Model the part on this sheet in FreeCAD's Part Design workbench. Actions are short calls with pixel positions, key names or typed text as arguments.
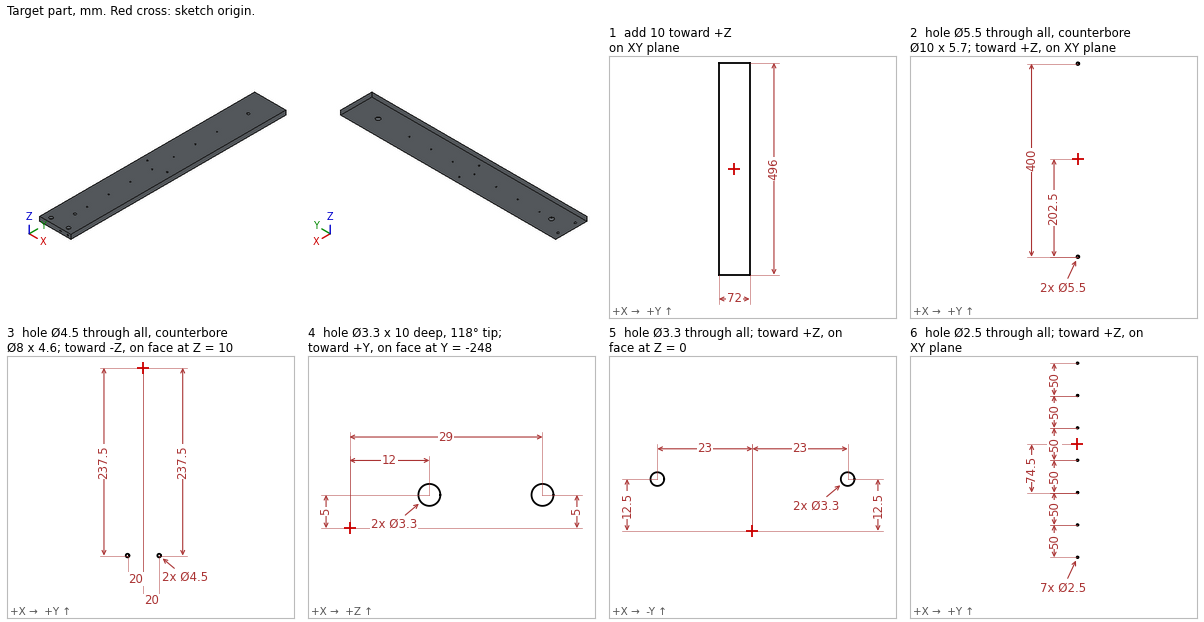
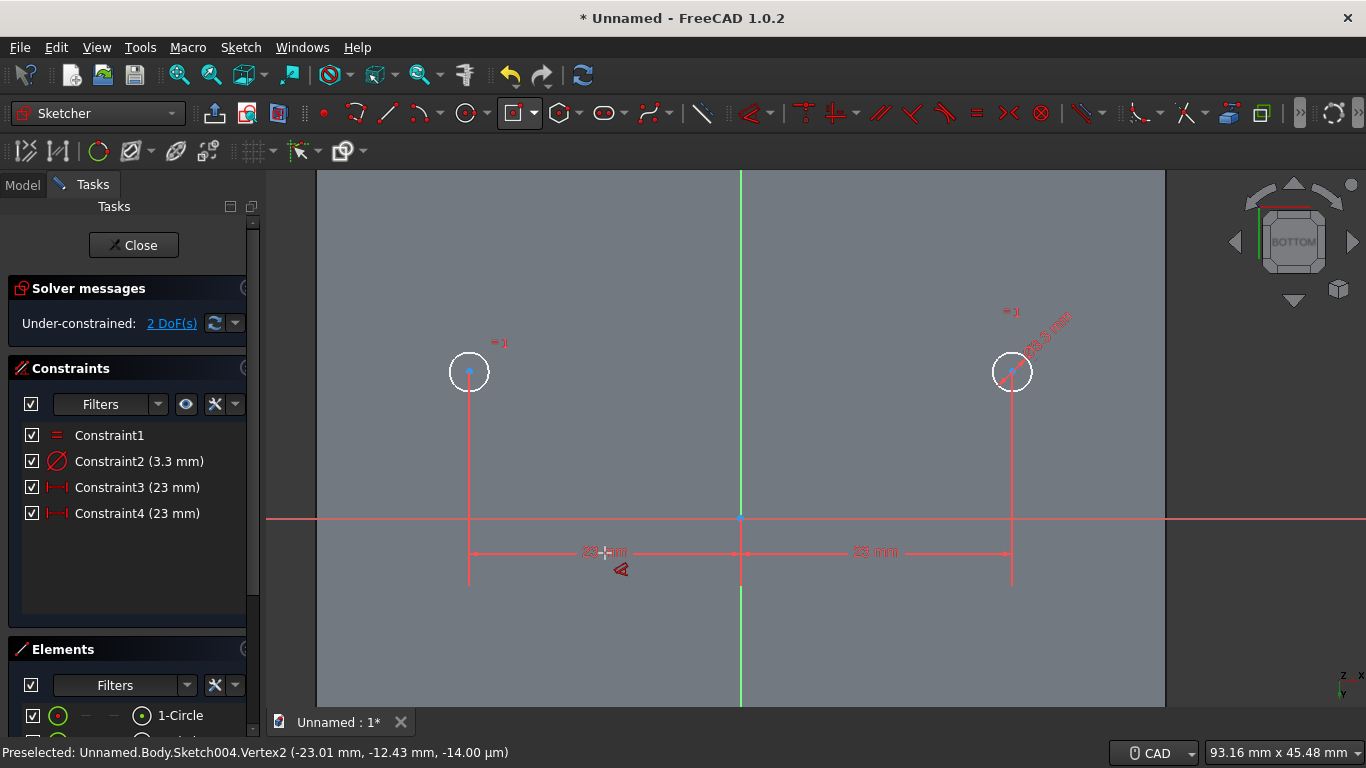
click(1012, 372)
click(1046, 445)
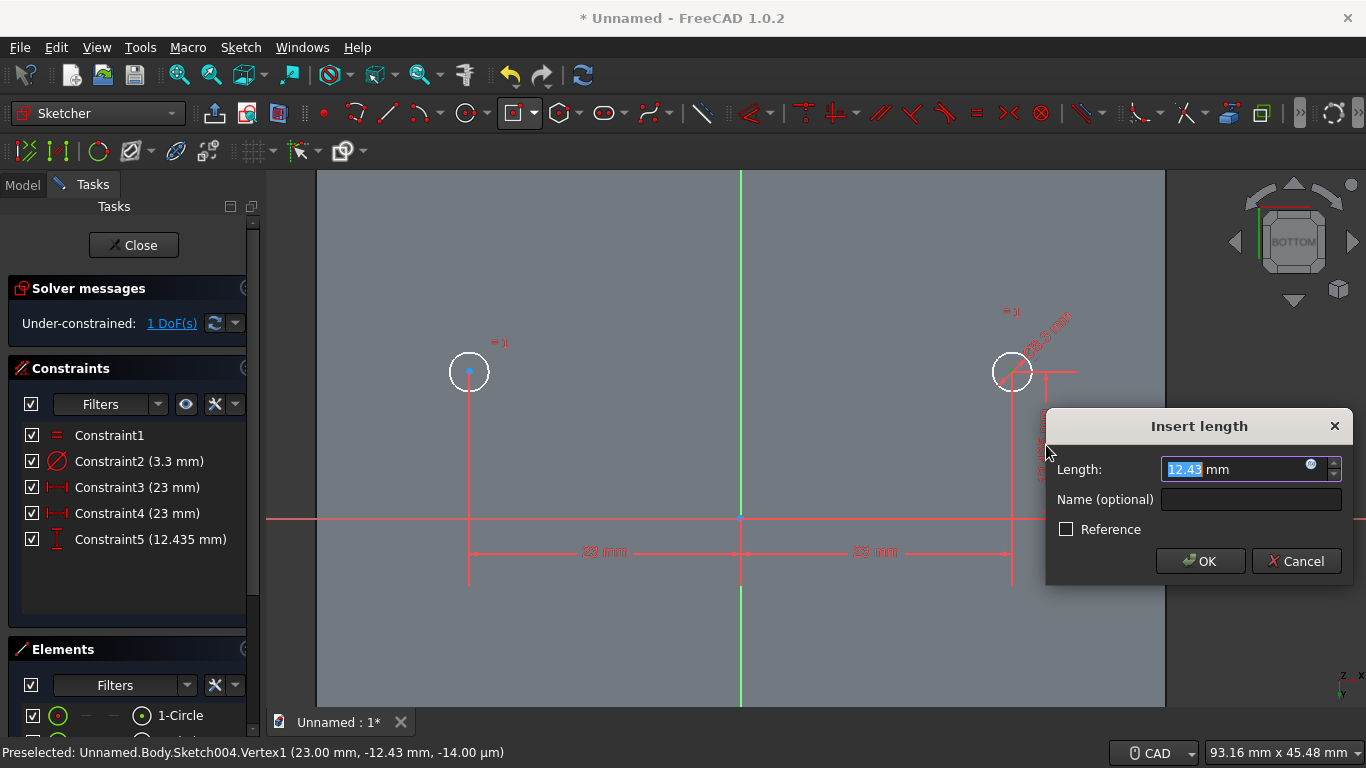
text(12.5)
key(Return)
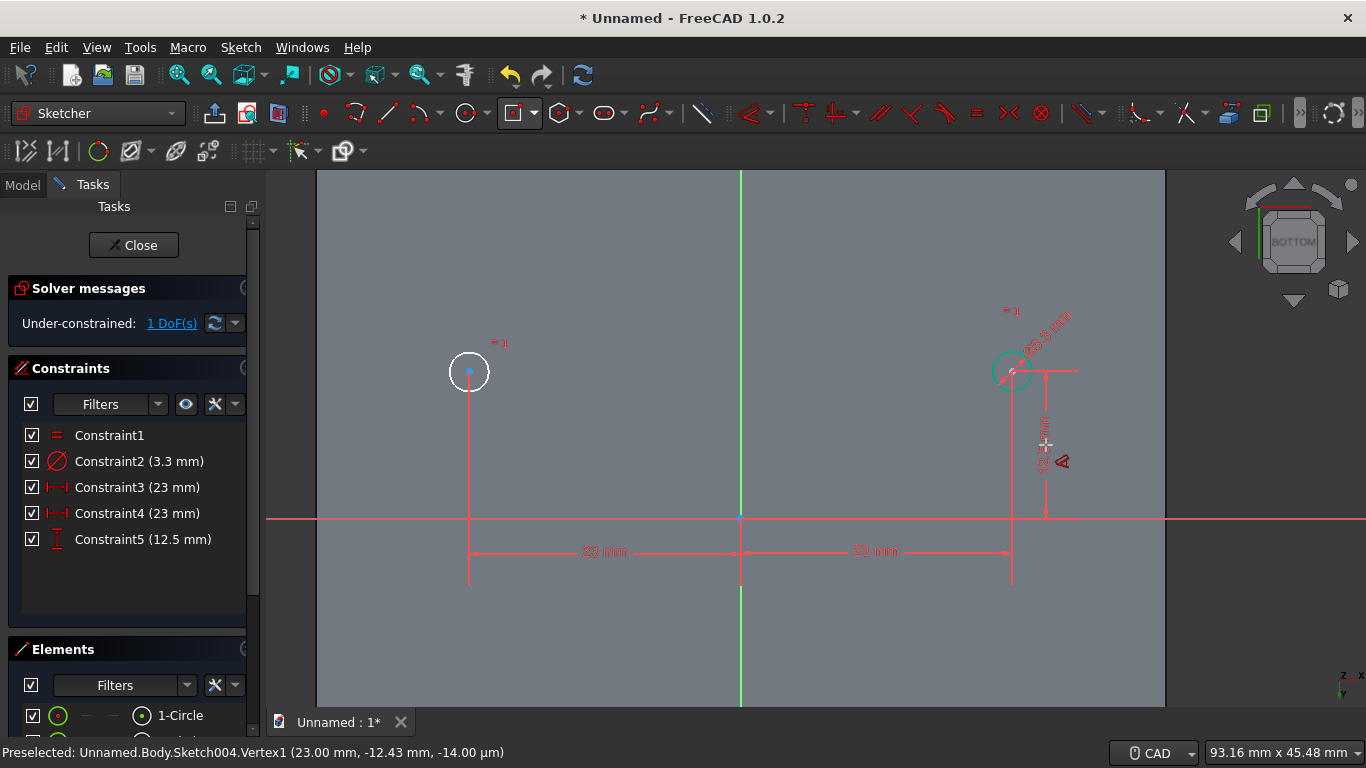
click(469, 372)
click(435, 445)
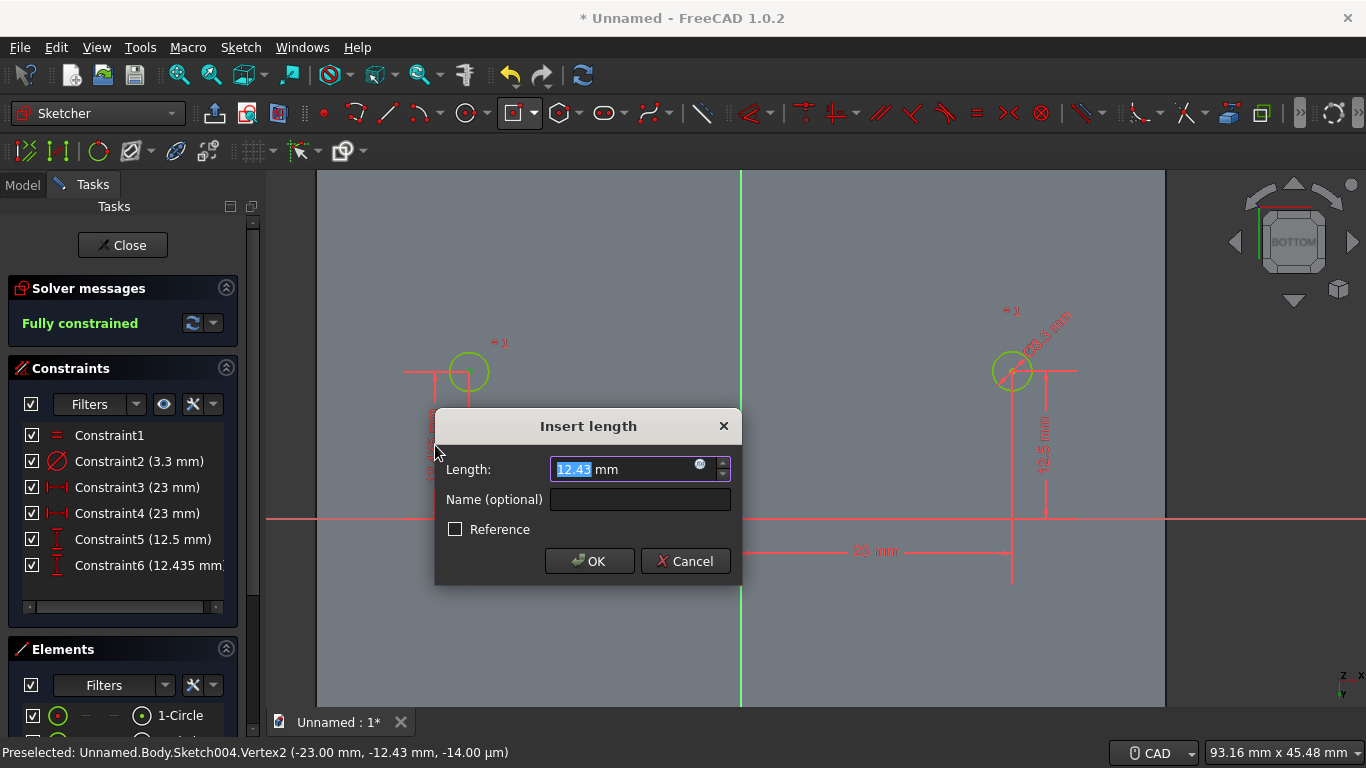
text(12.5)
key(Return)
key(Escape)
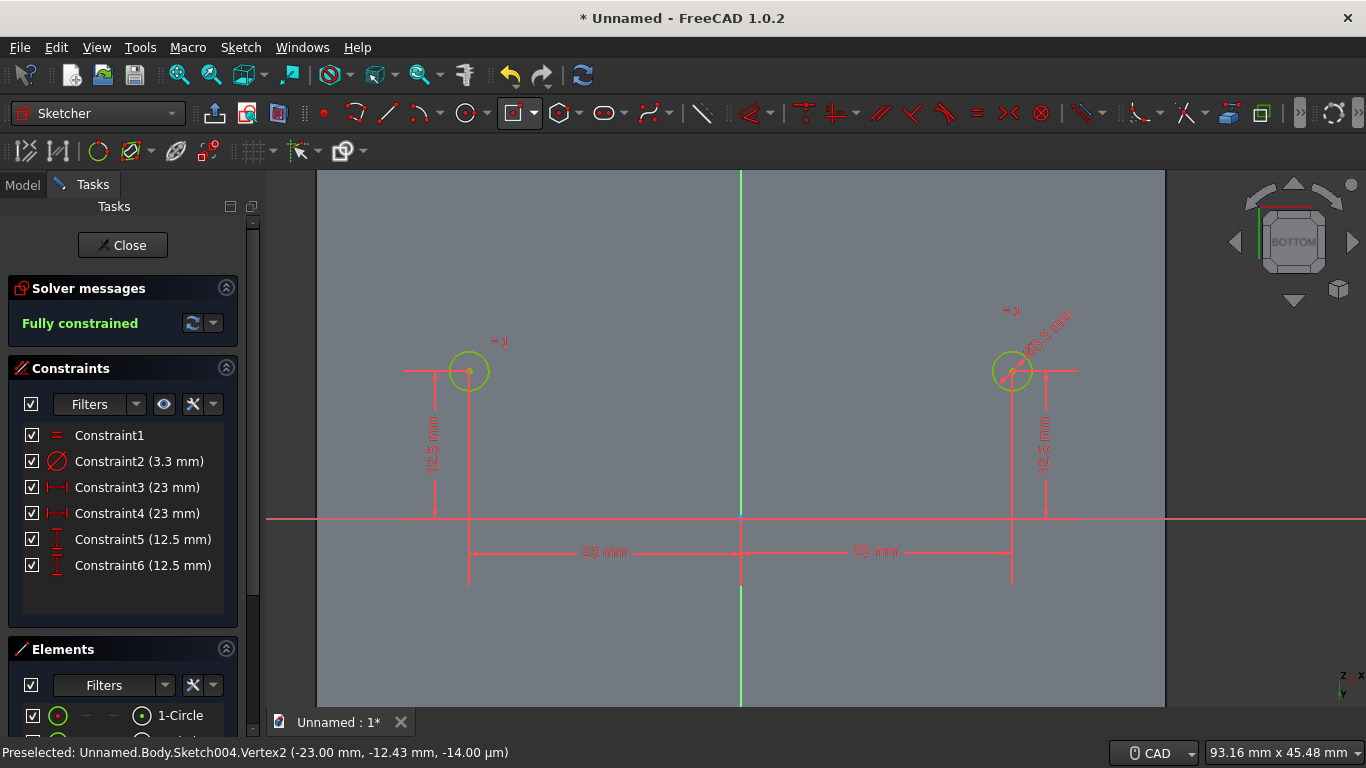
click(123, 245)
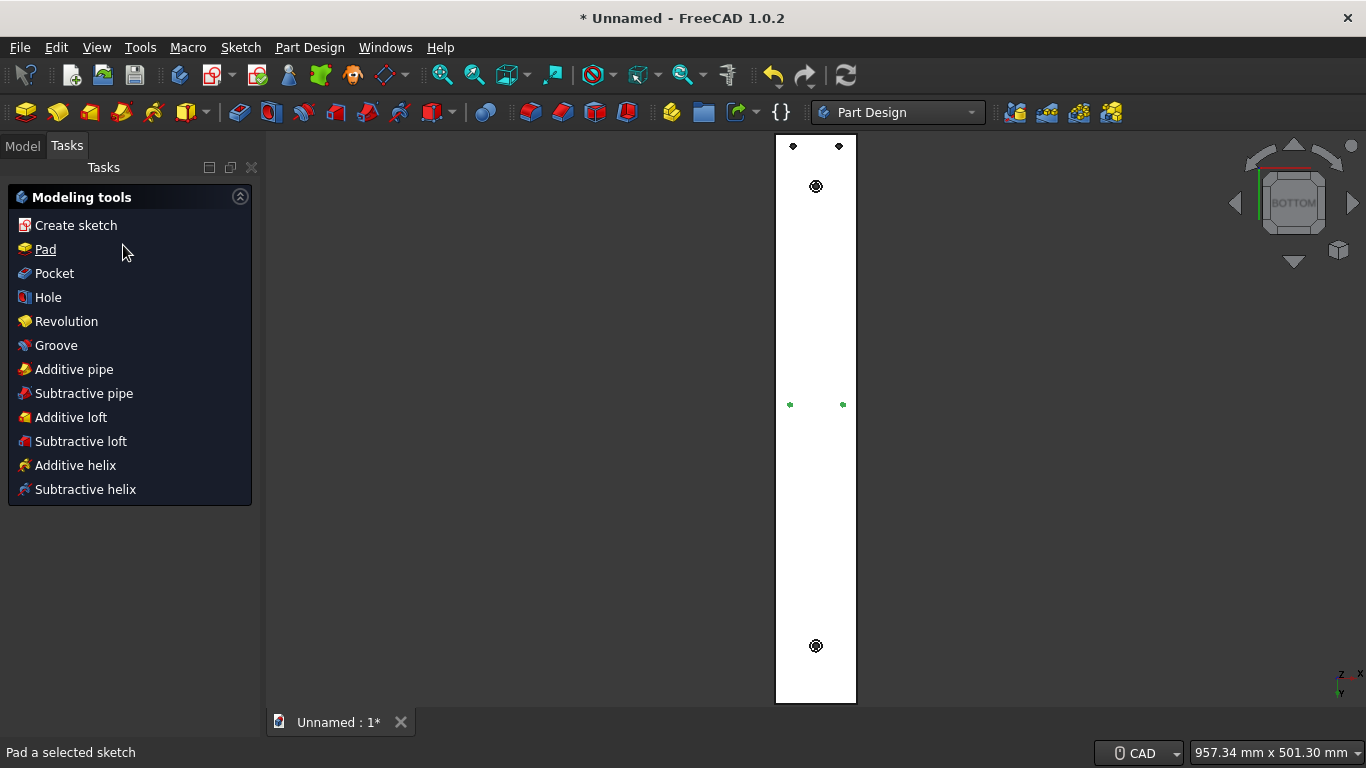
click(272, 112)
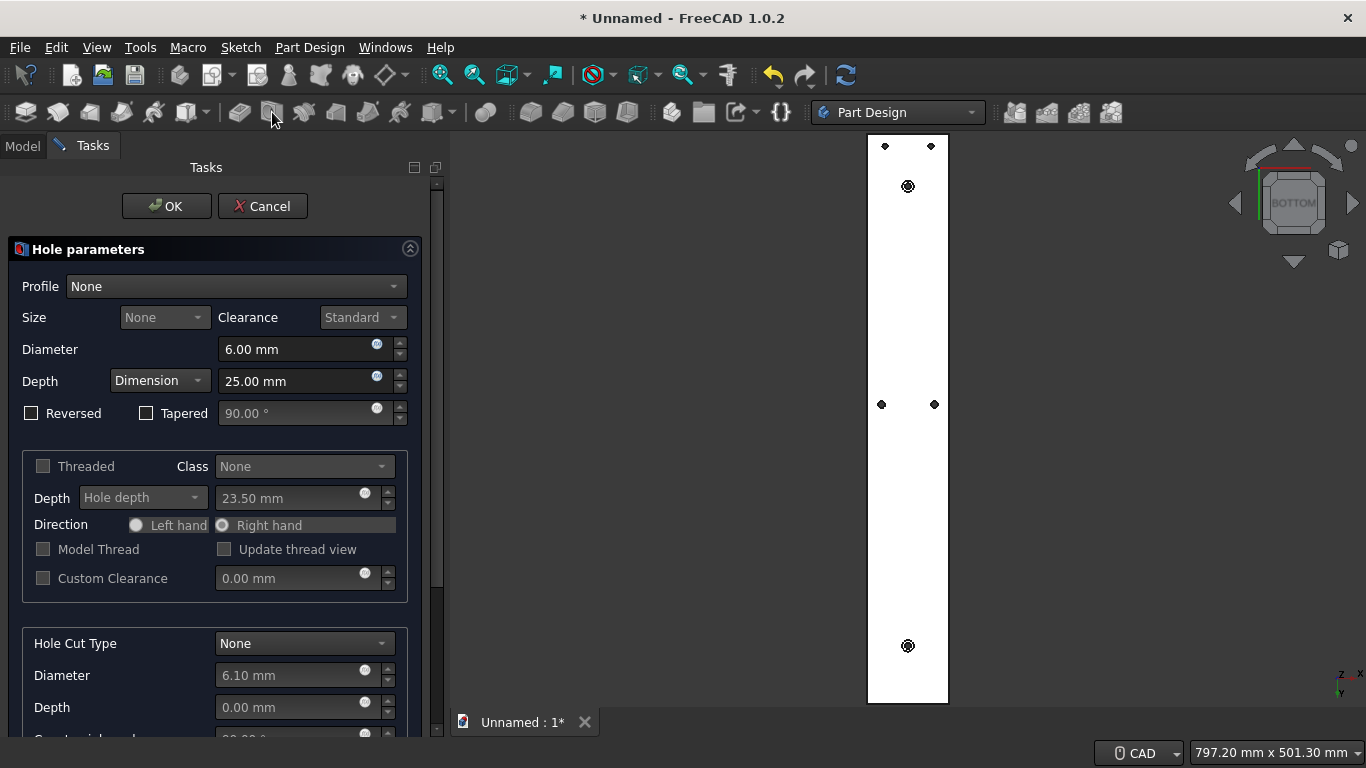
triple_click(305, 349)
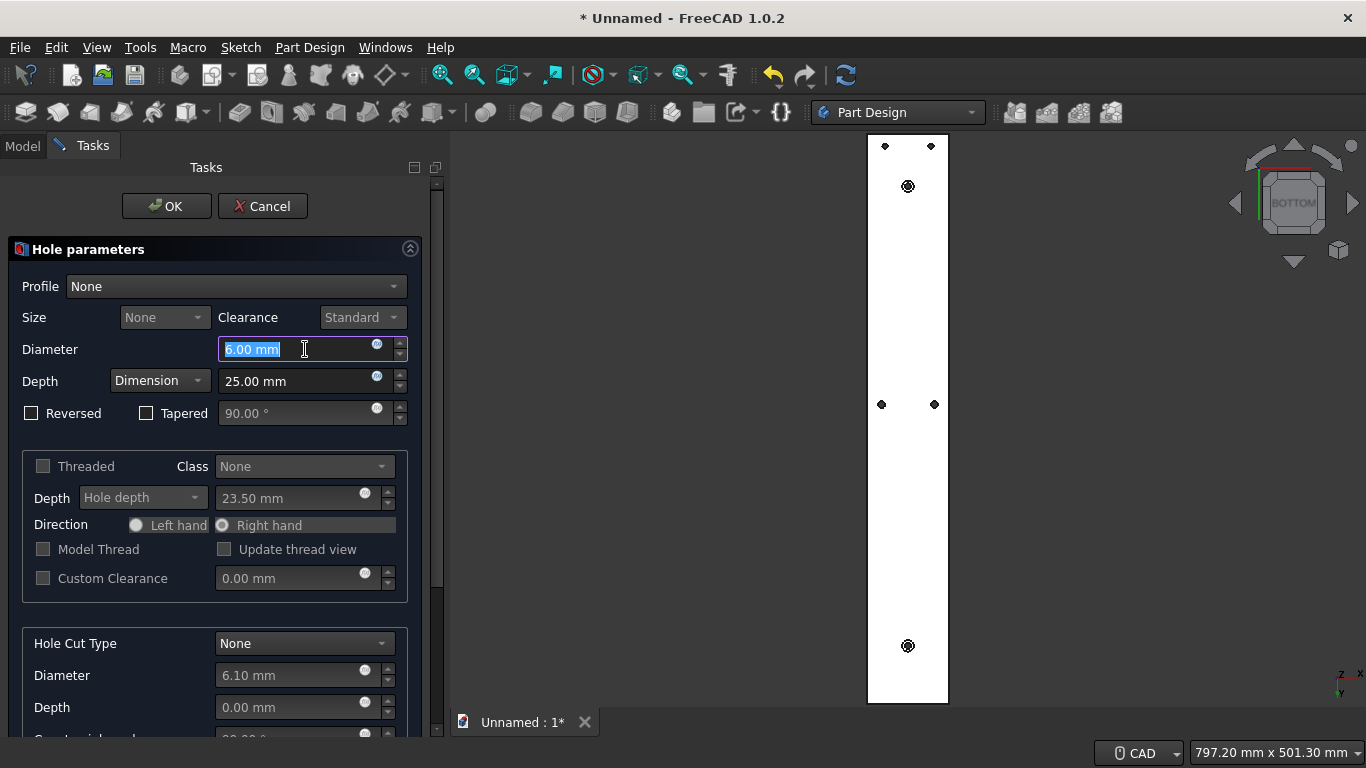
text(3.3)
key(Tab)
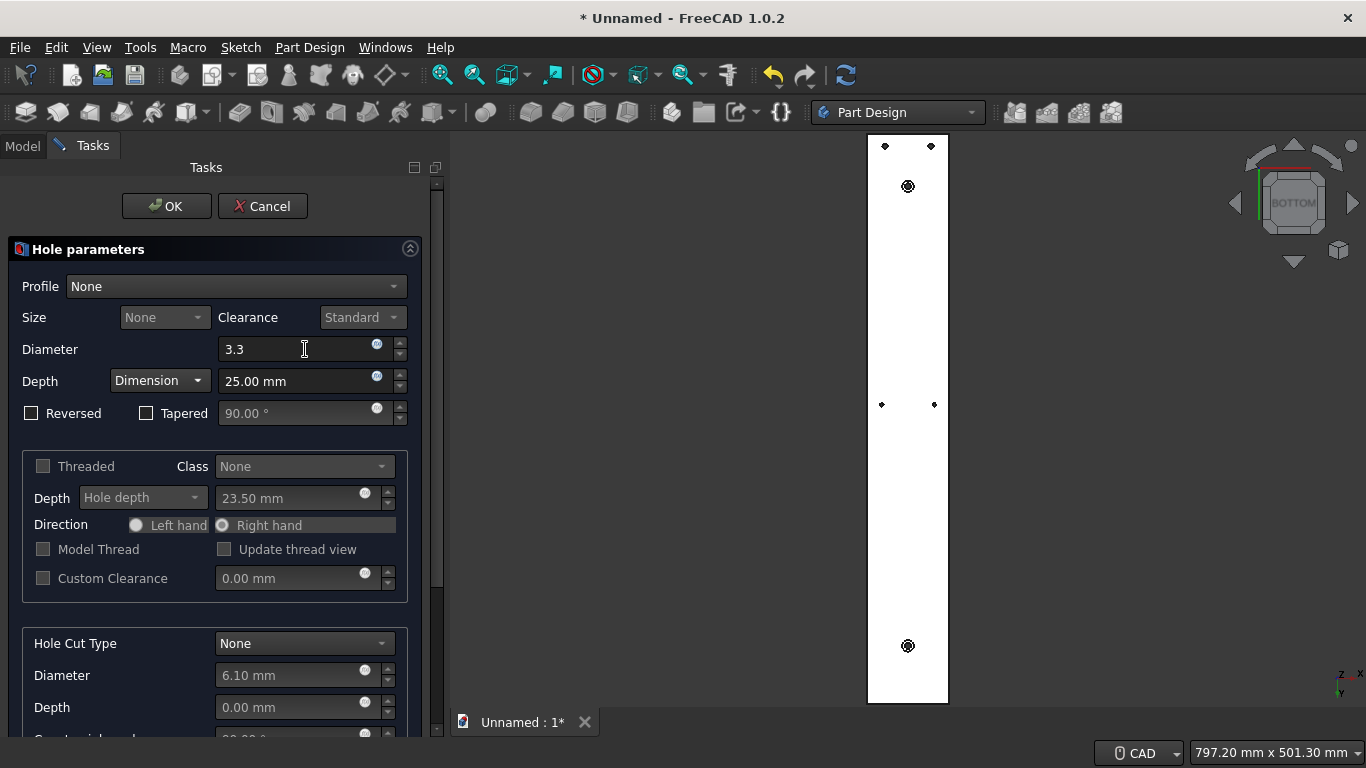
click(161, 380)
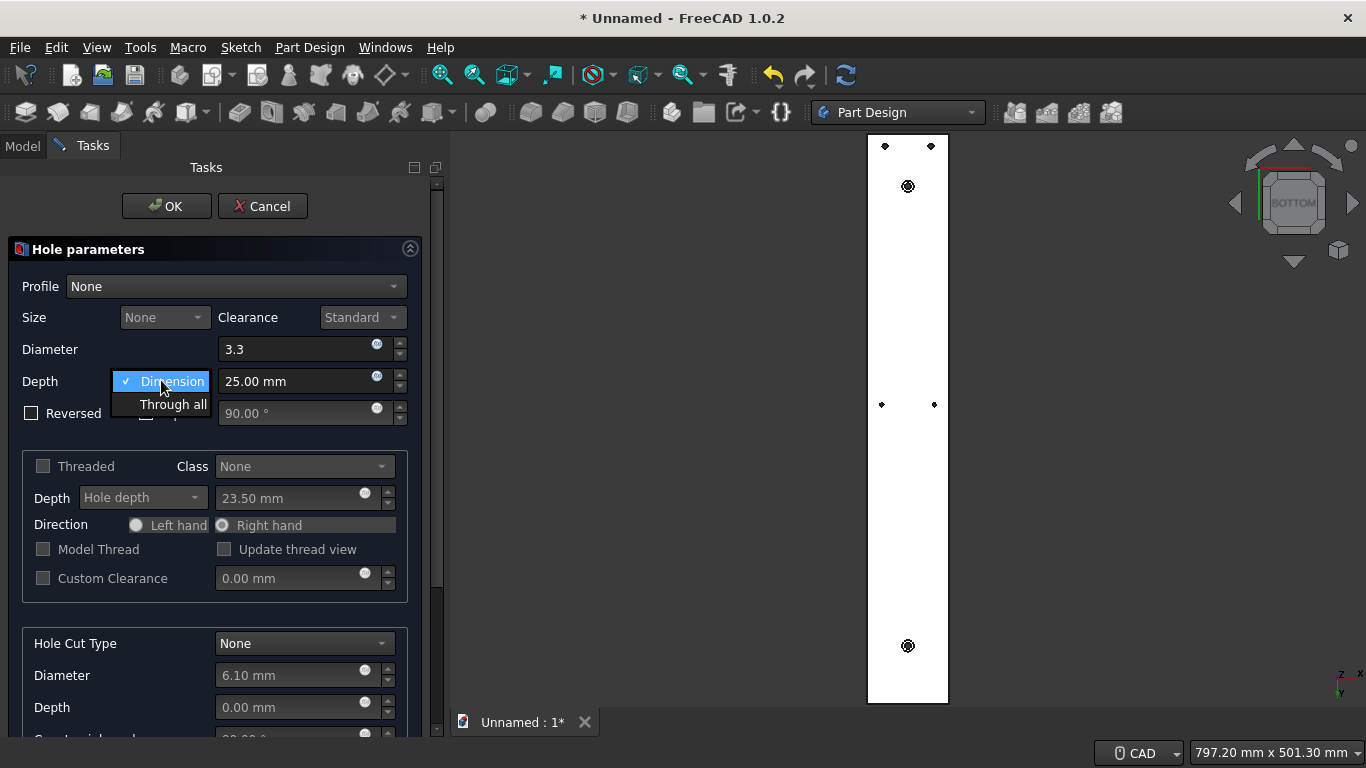
click(160, 404)